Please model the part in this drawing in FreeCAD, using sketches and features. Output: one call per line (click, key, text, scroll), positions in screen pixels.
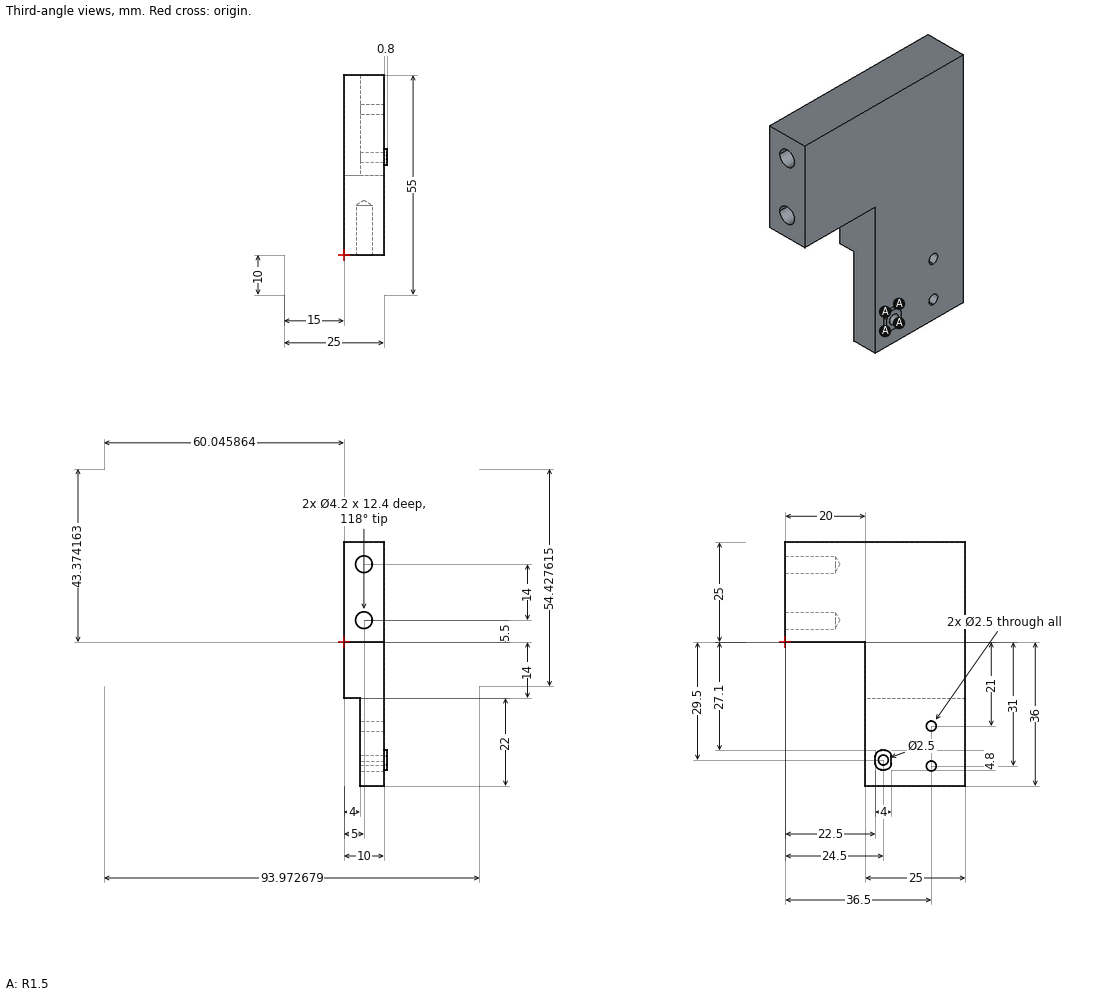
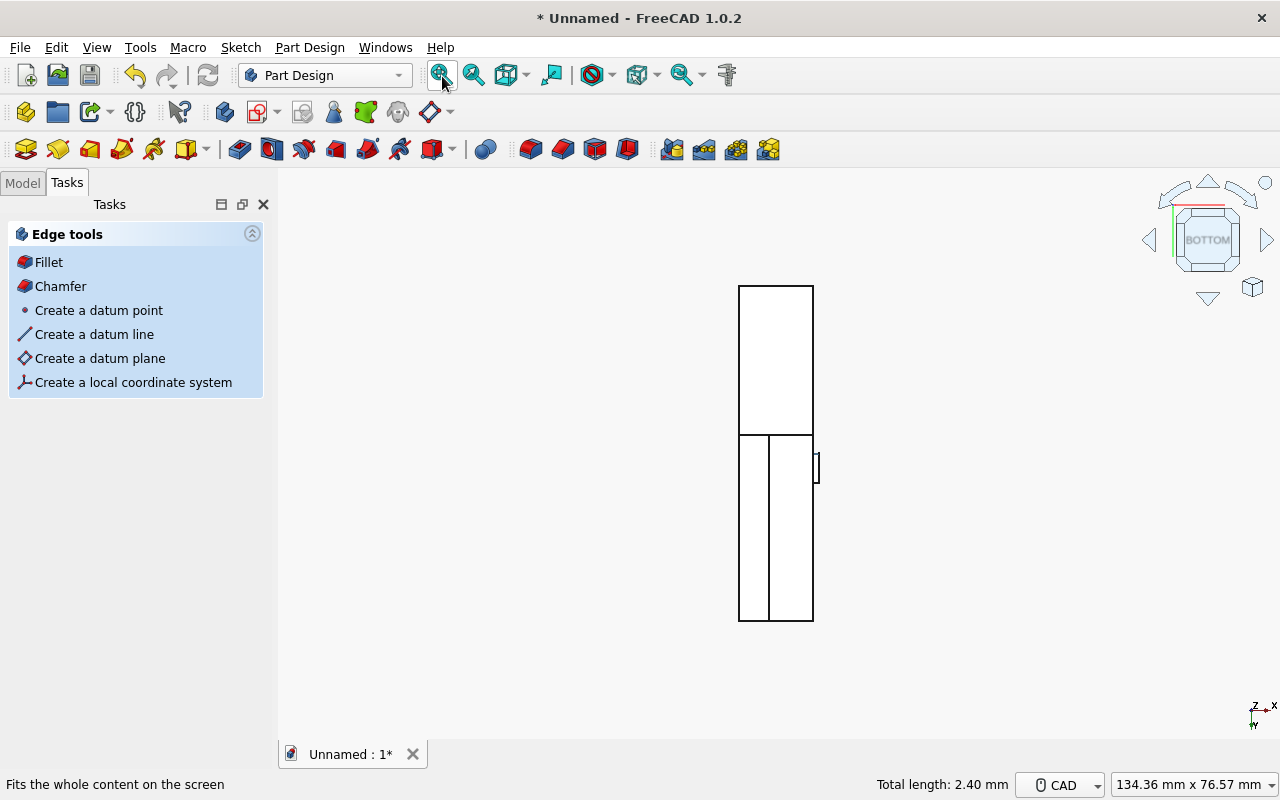
scroll(816, 482, up, 10)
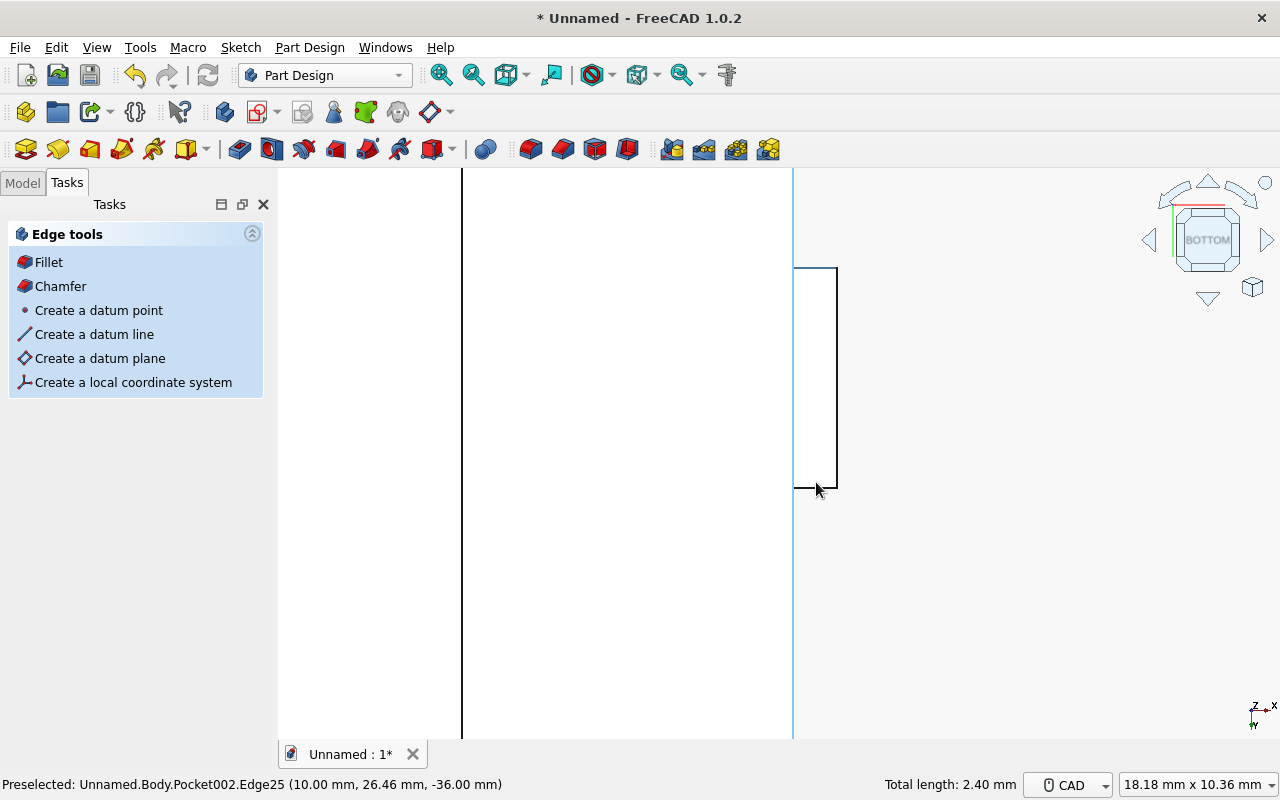
click(815, 487, ctrl)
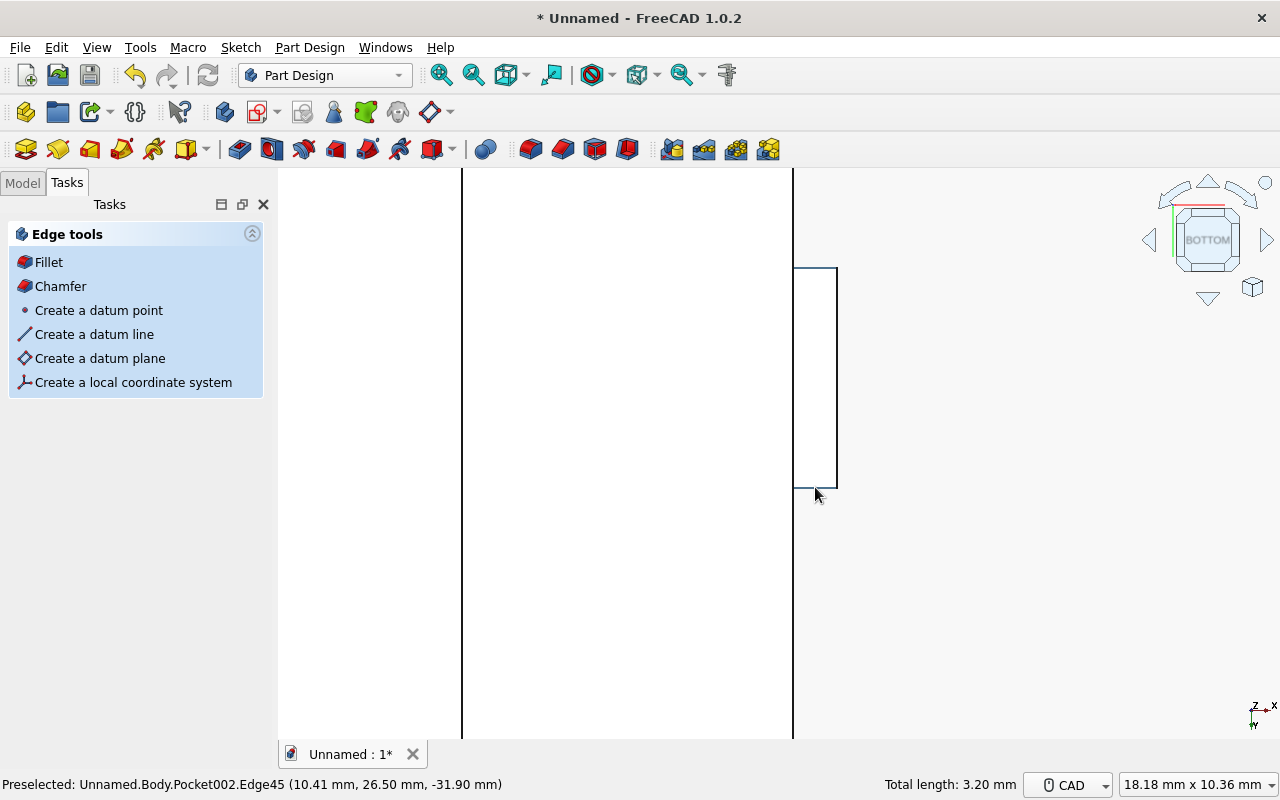
click(532, 150)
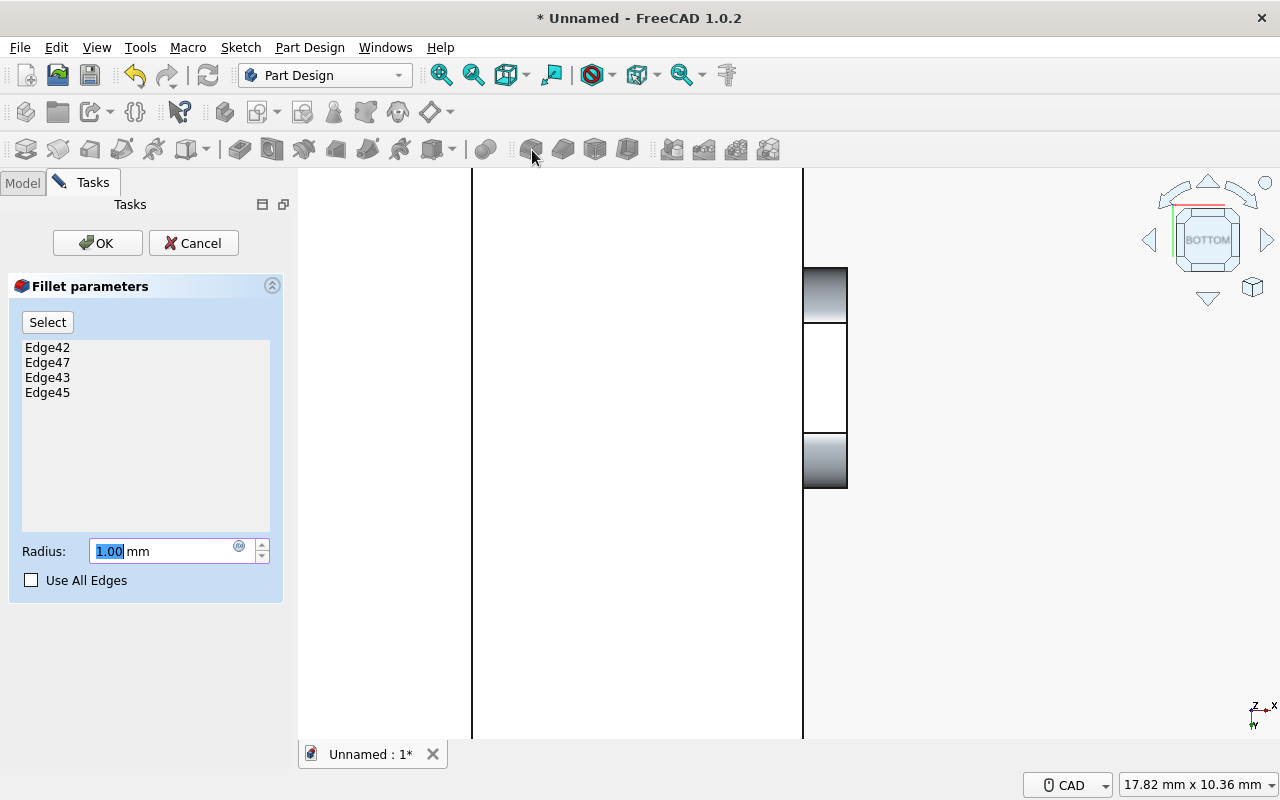
text(1.5)
key(Tab)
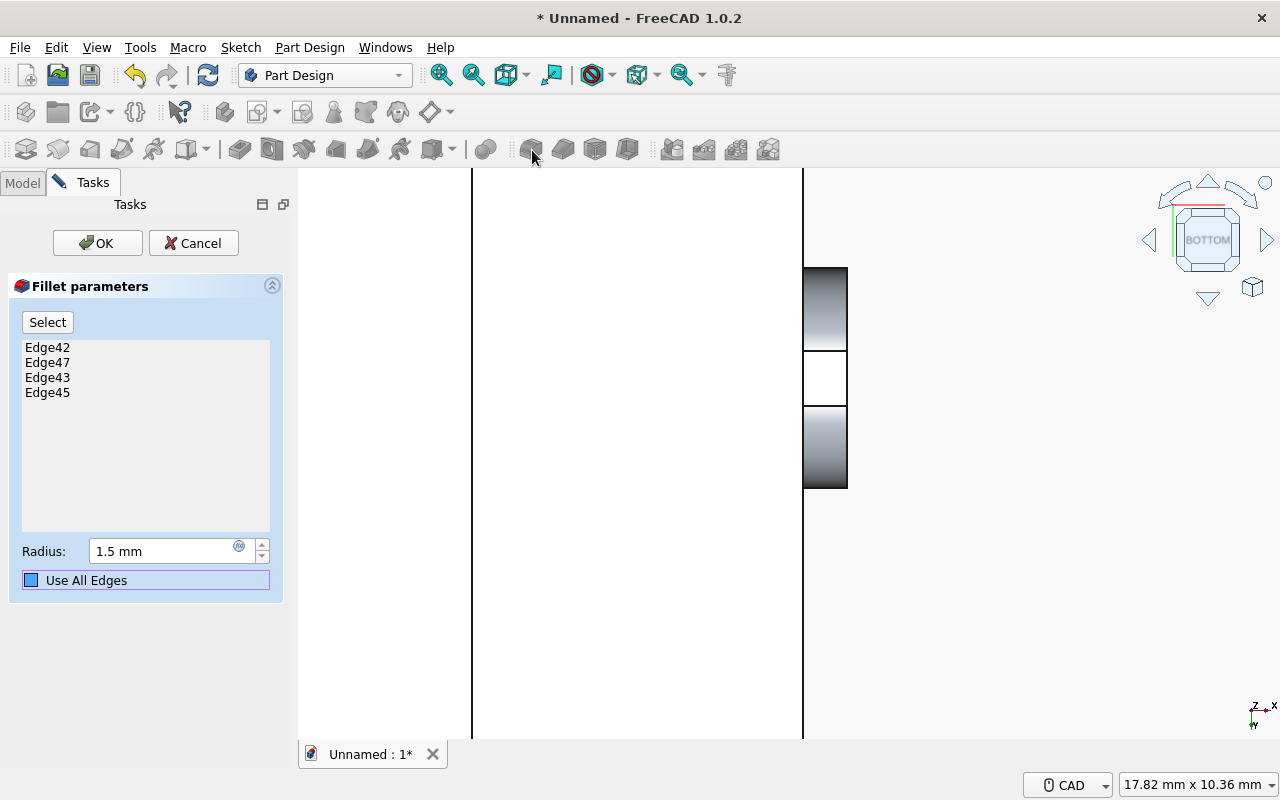
click(98, 243)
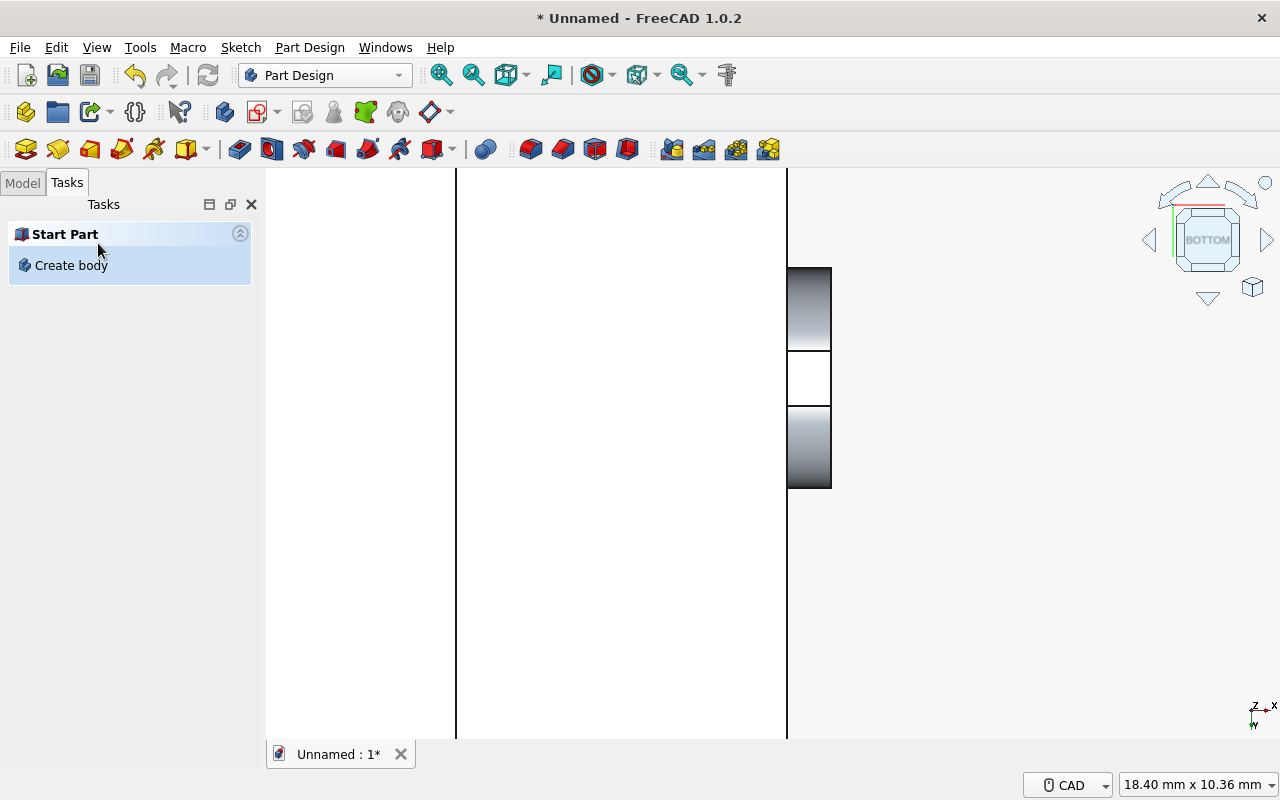
key(0)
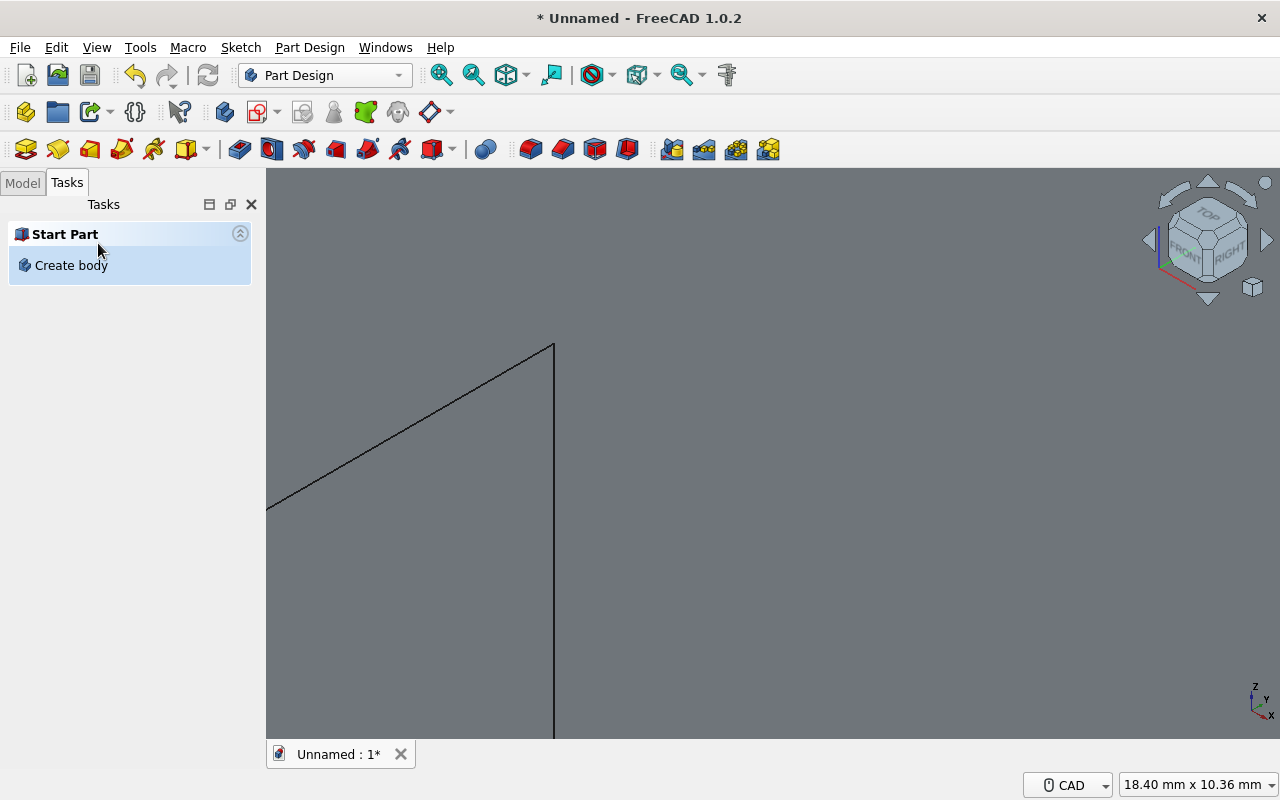
click(442, 76)